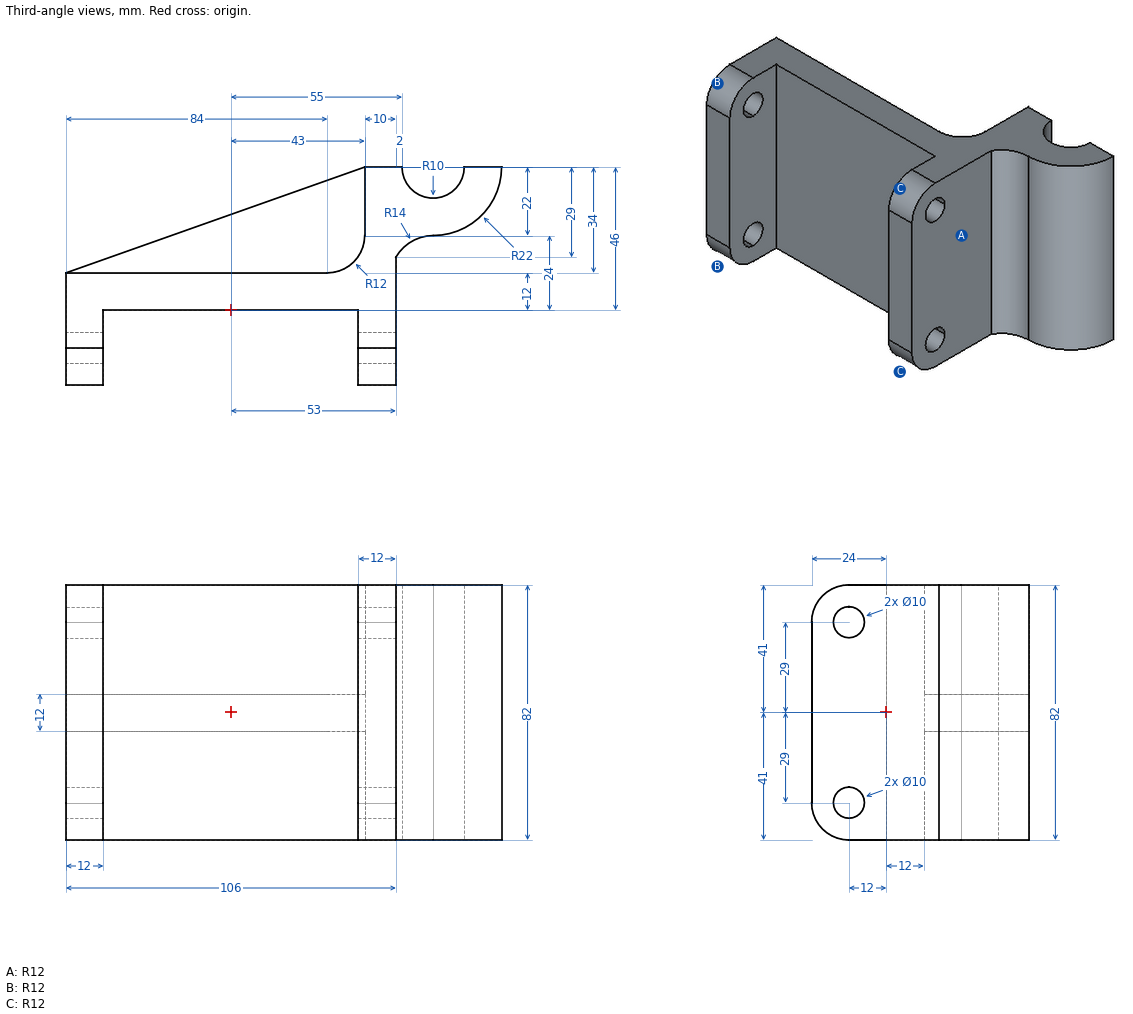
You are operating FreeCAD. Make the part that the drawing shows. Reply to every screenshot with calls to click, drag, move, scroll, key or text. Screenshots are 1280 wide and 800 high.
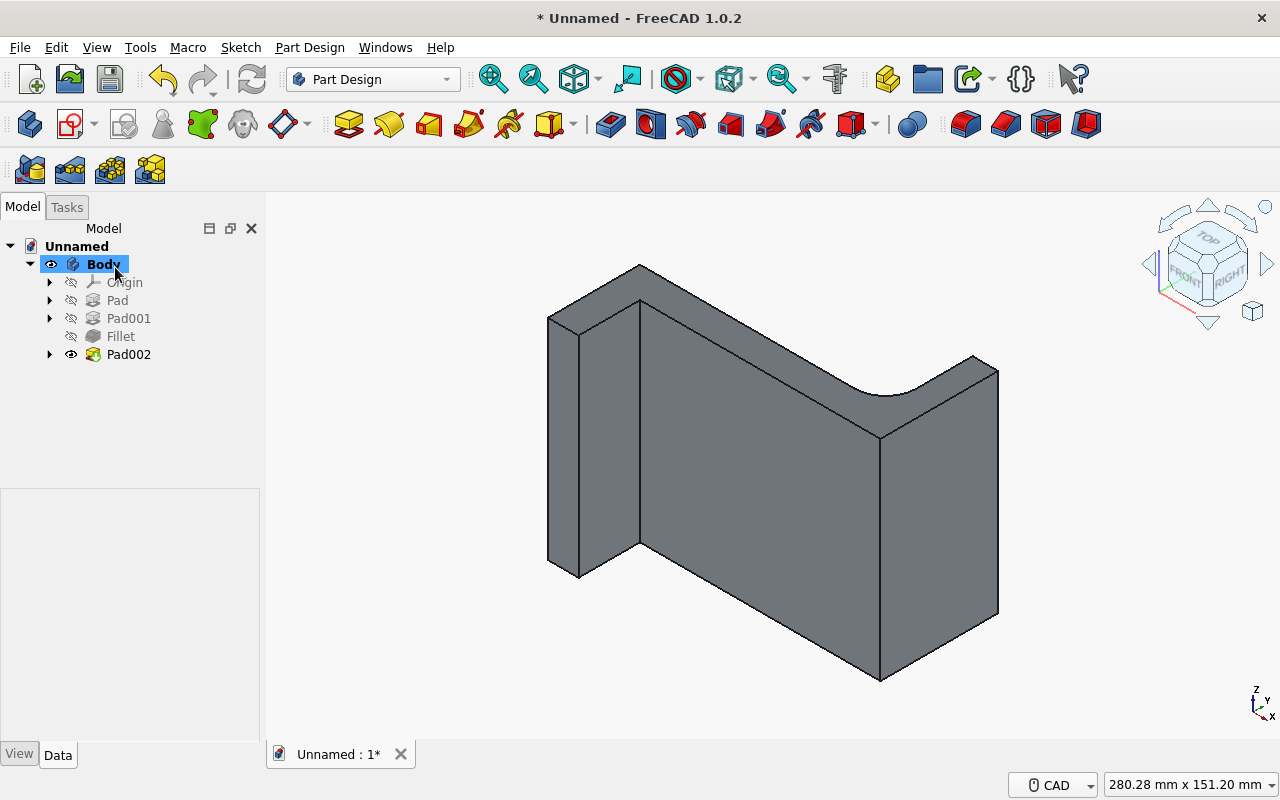
click(563, 326)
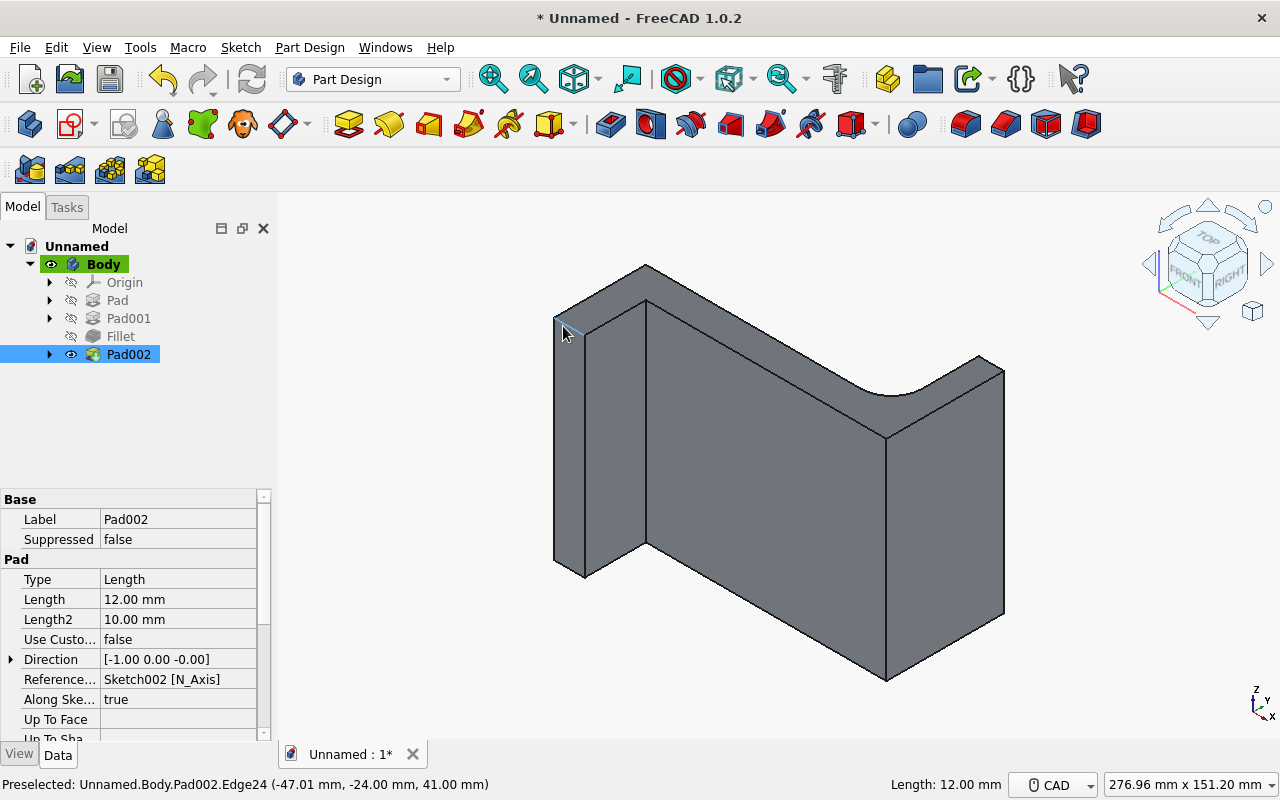
key(2)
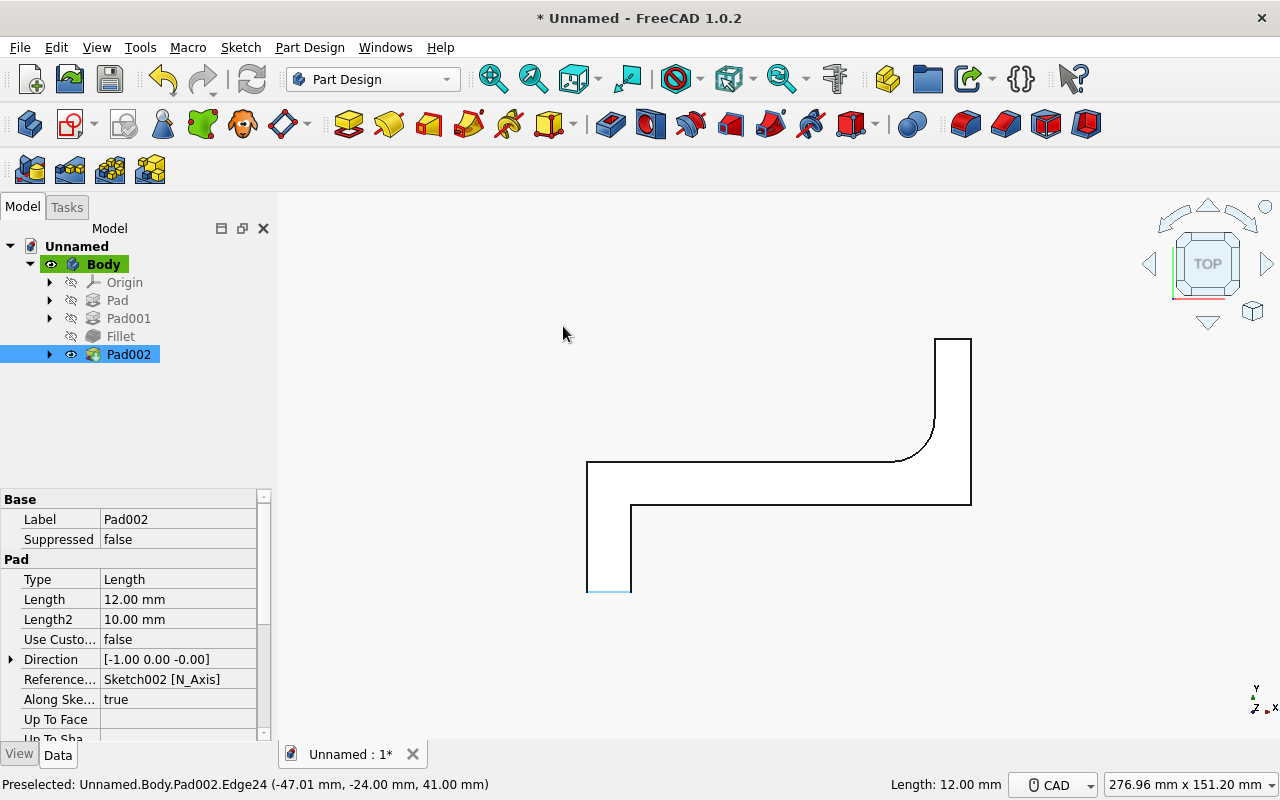
key(1)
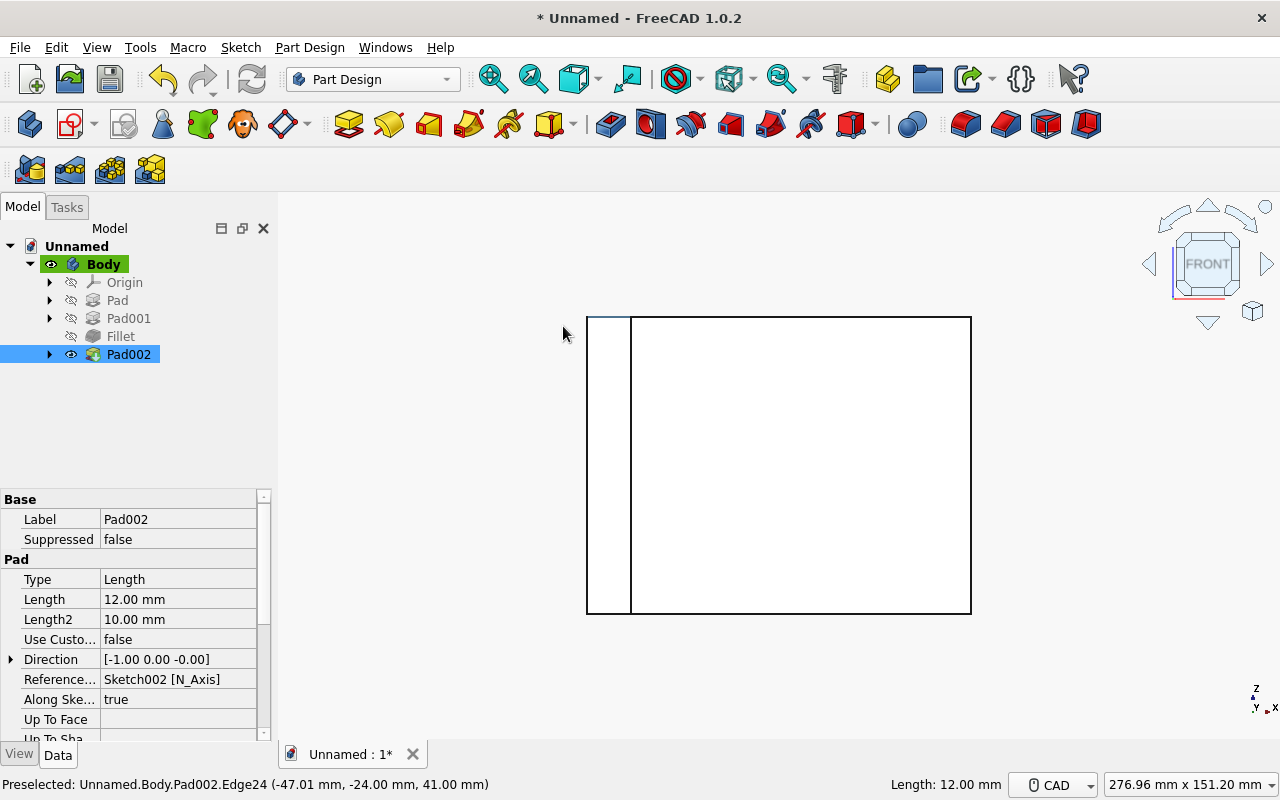
key(3)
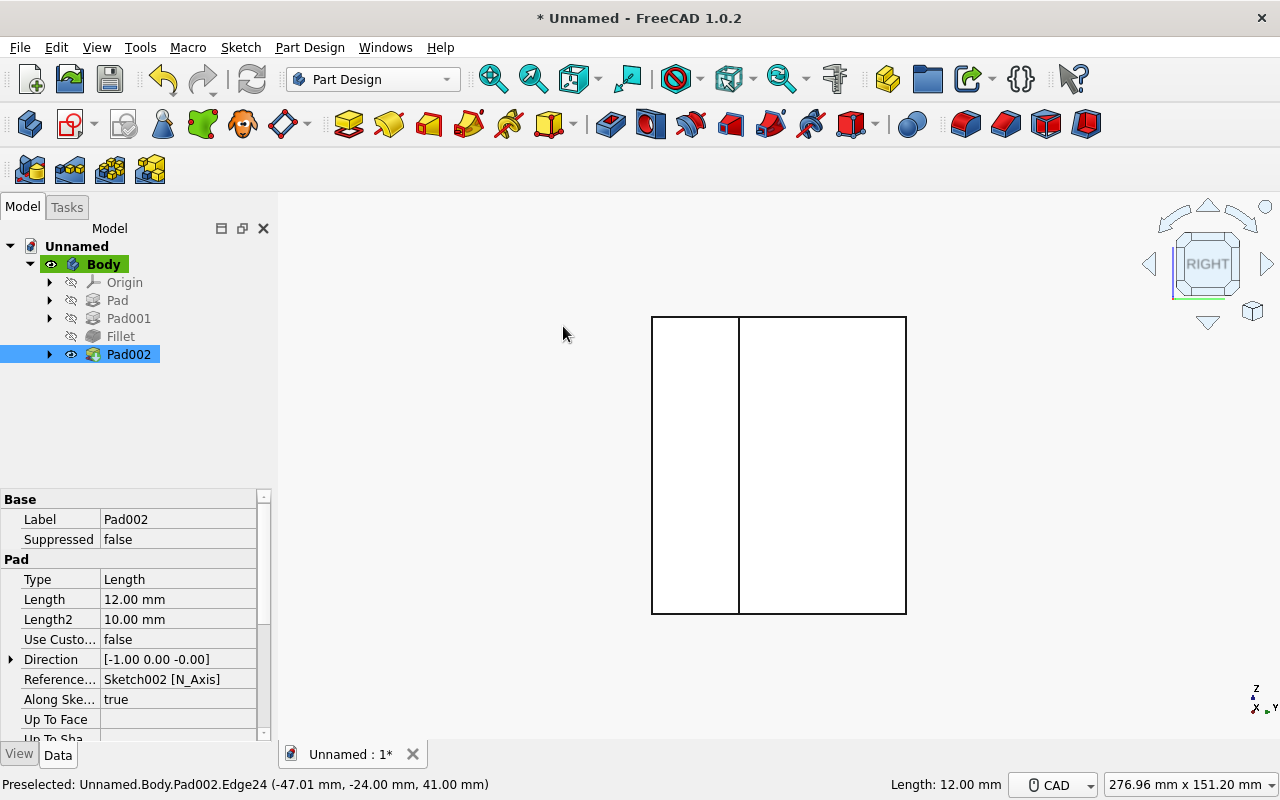
key(5)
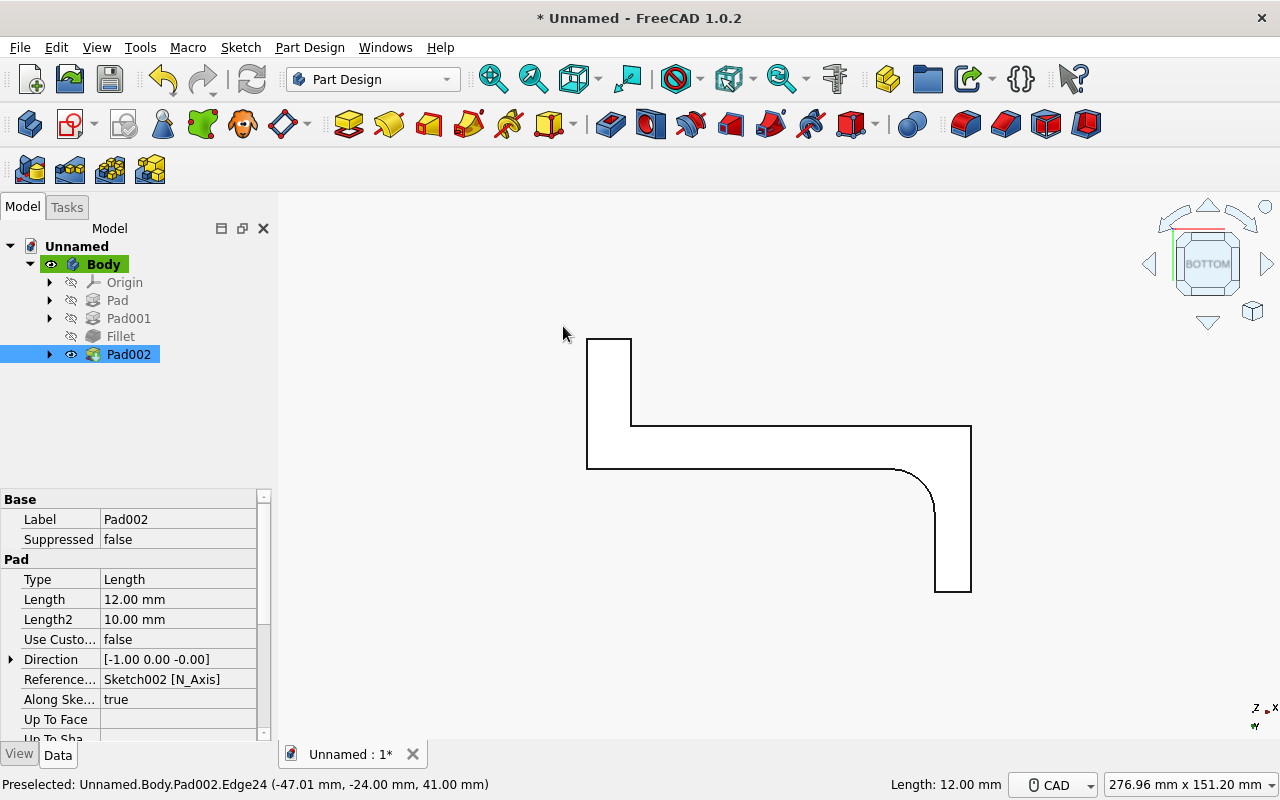
click(609, 338, ctrl)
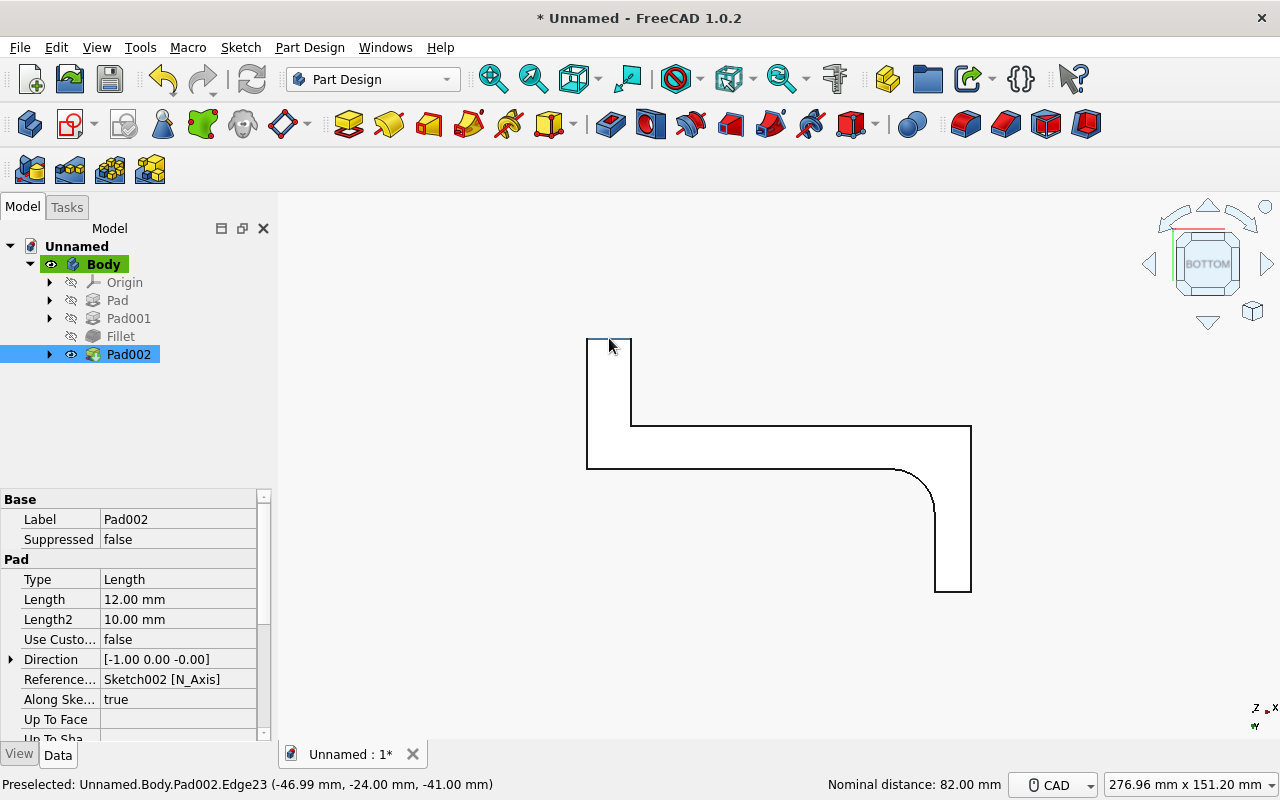
click(966, 124)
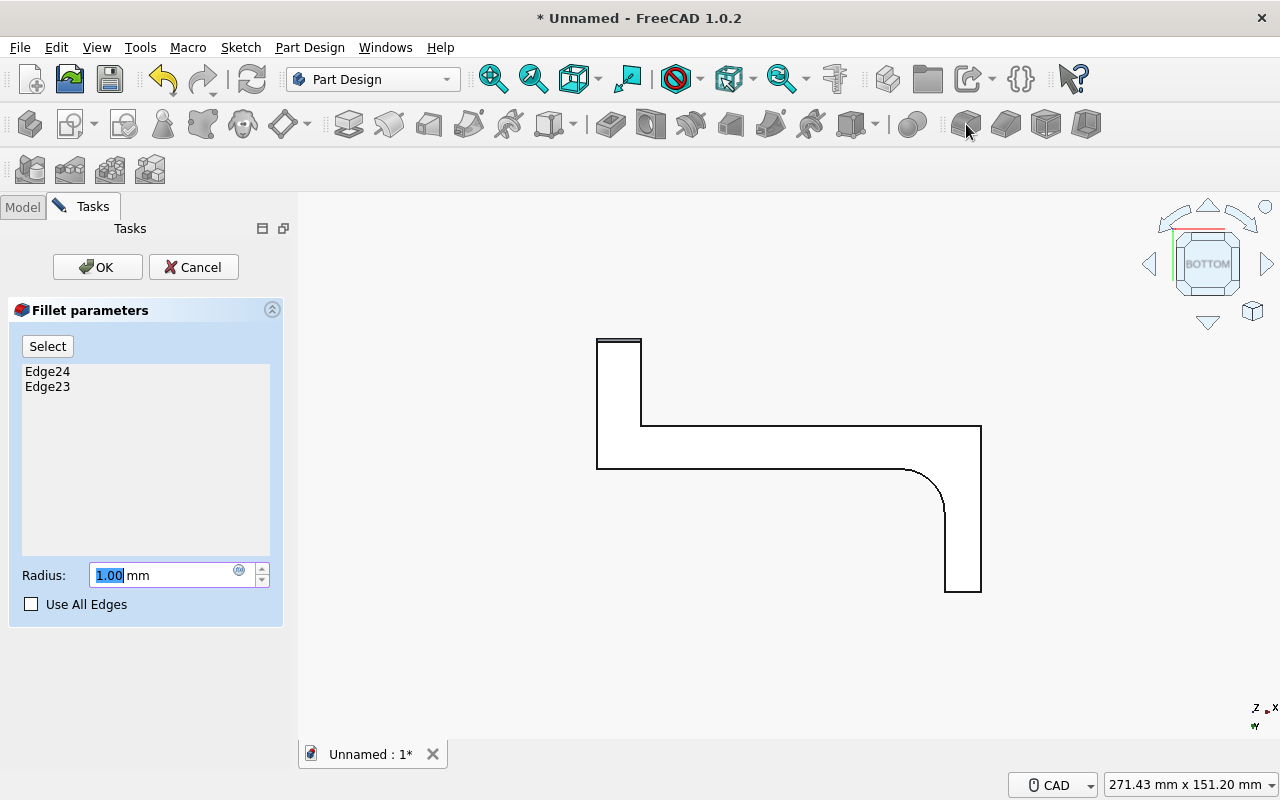
text(12)
key(Tab)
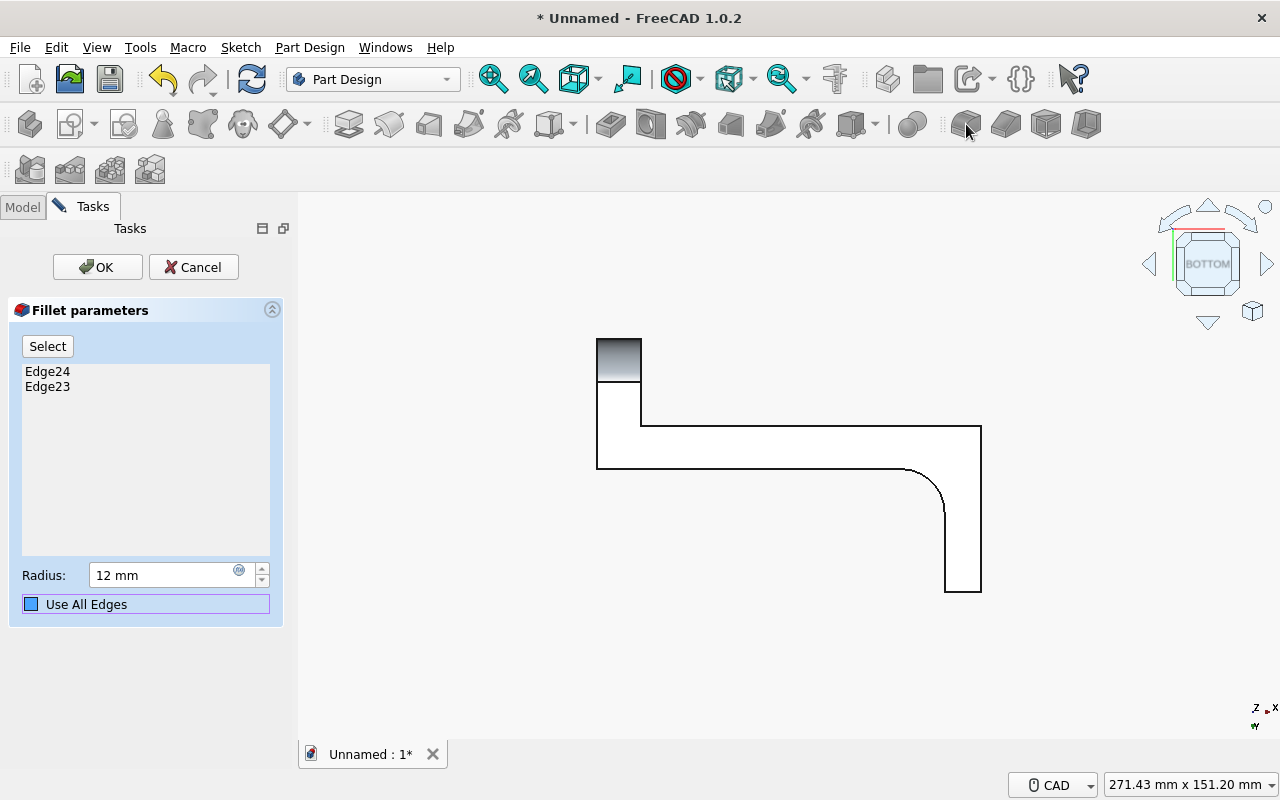
click(98, 267)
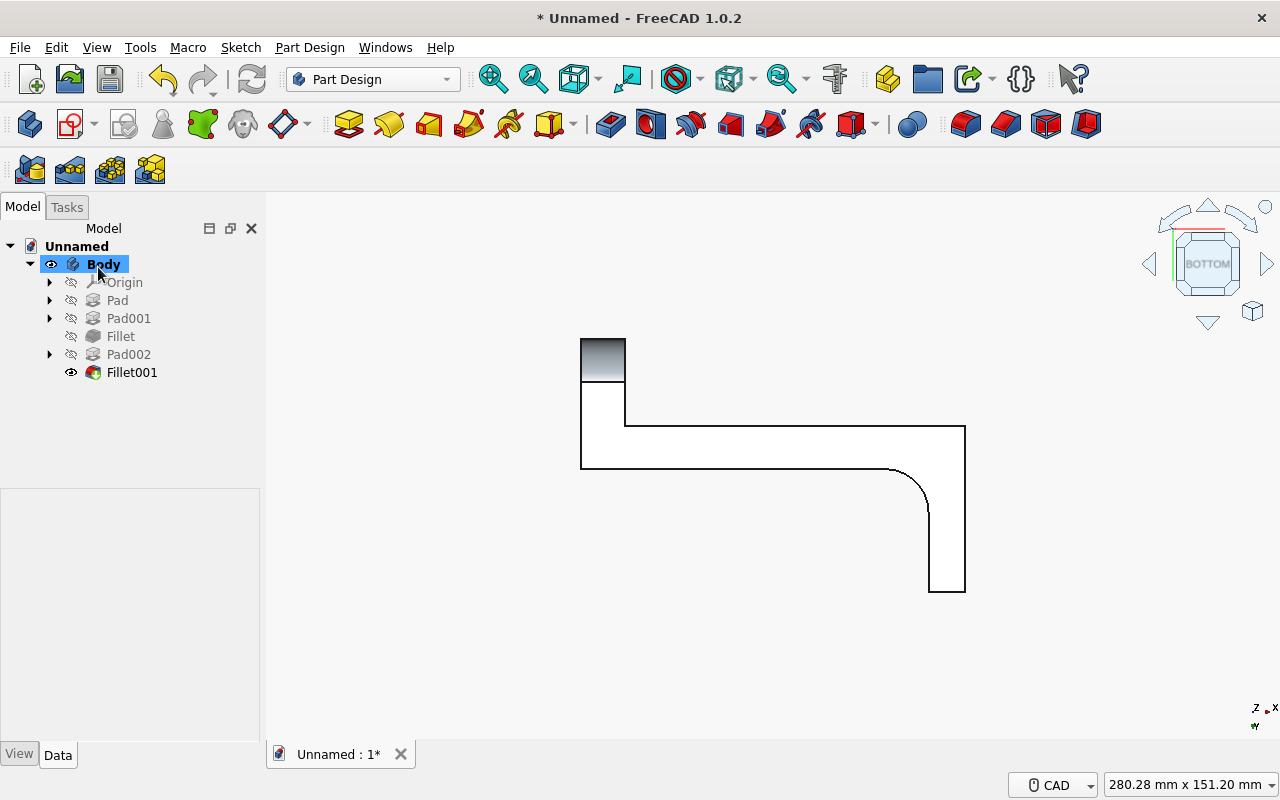
key(6)